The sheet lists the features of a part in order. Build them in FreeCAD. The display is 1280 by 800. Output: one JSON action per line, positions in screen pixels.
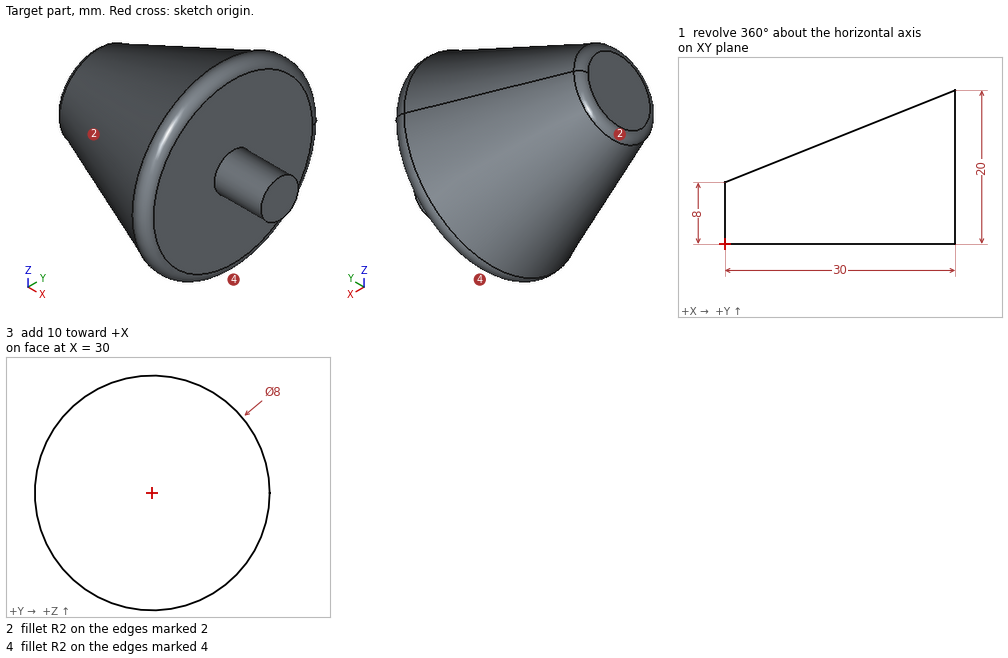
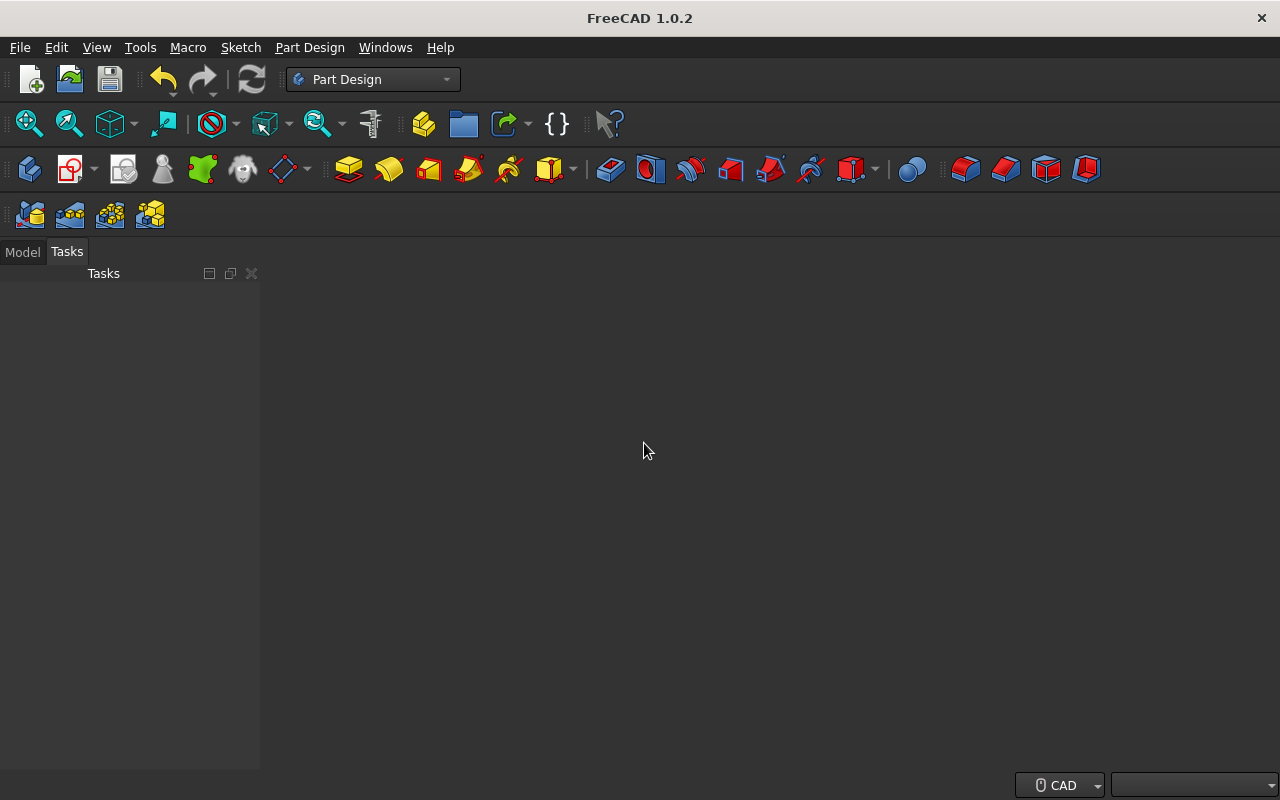
{"action": "left_click", "coordinate": [30, 80]}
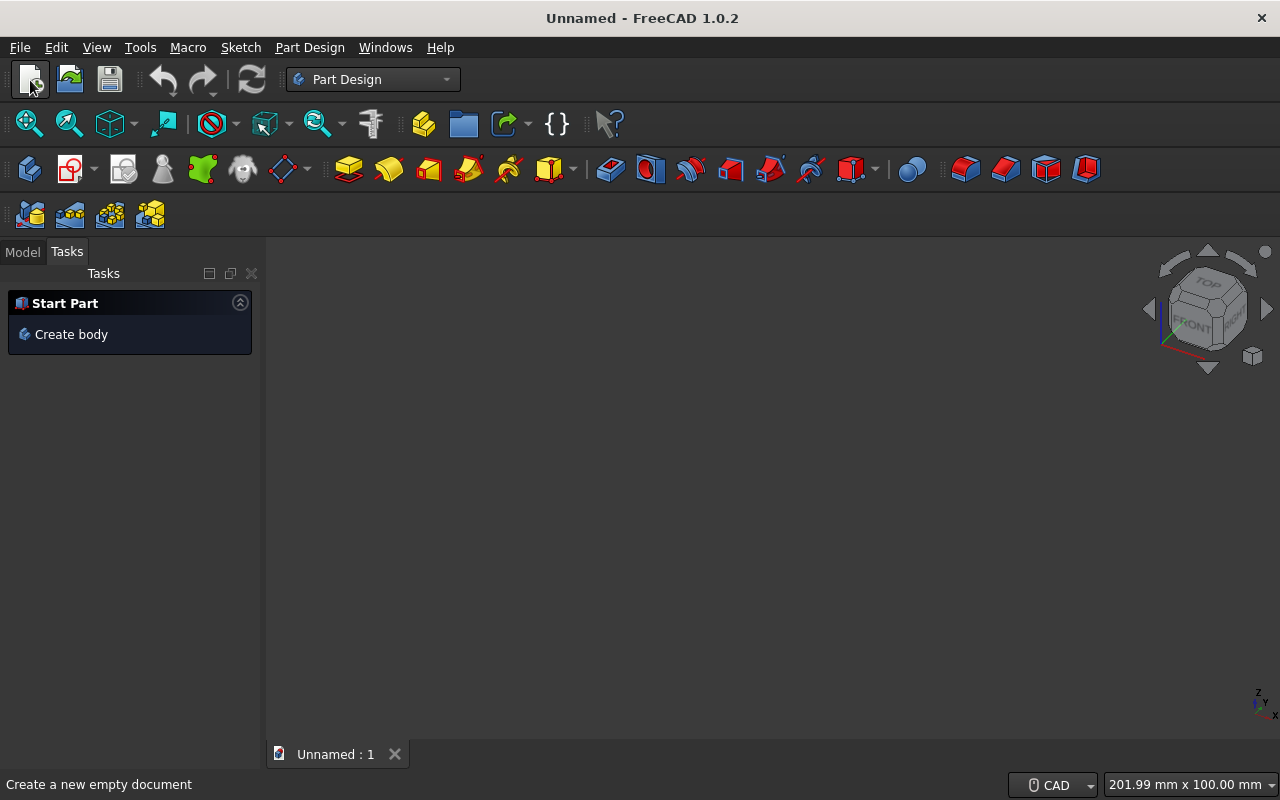
{"action": "left_click", "coordinate": [70, 170]}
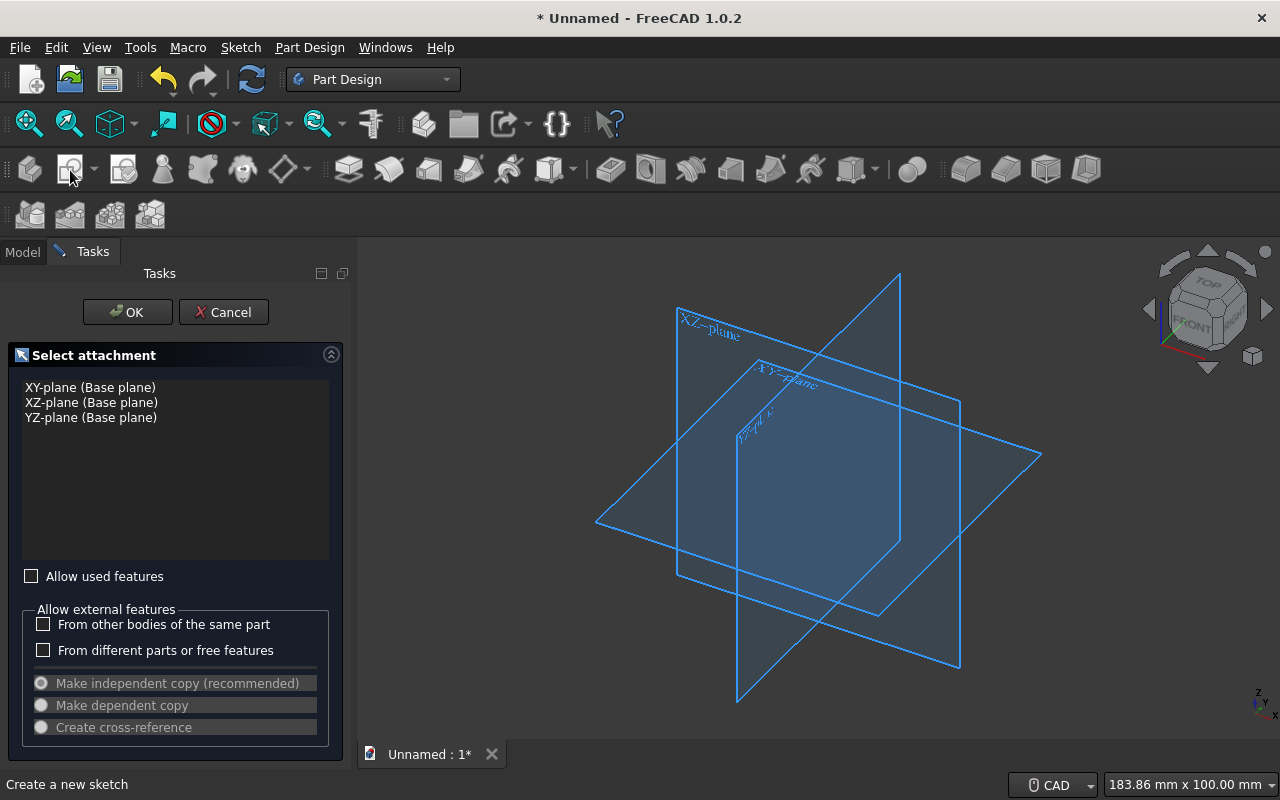
{"action": "left_click", "coordinate": [82, 388]}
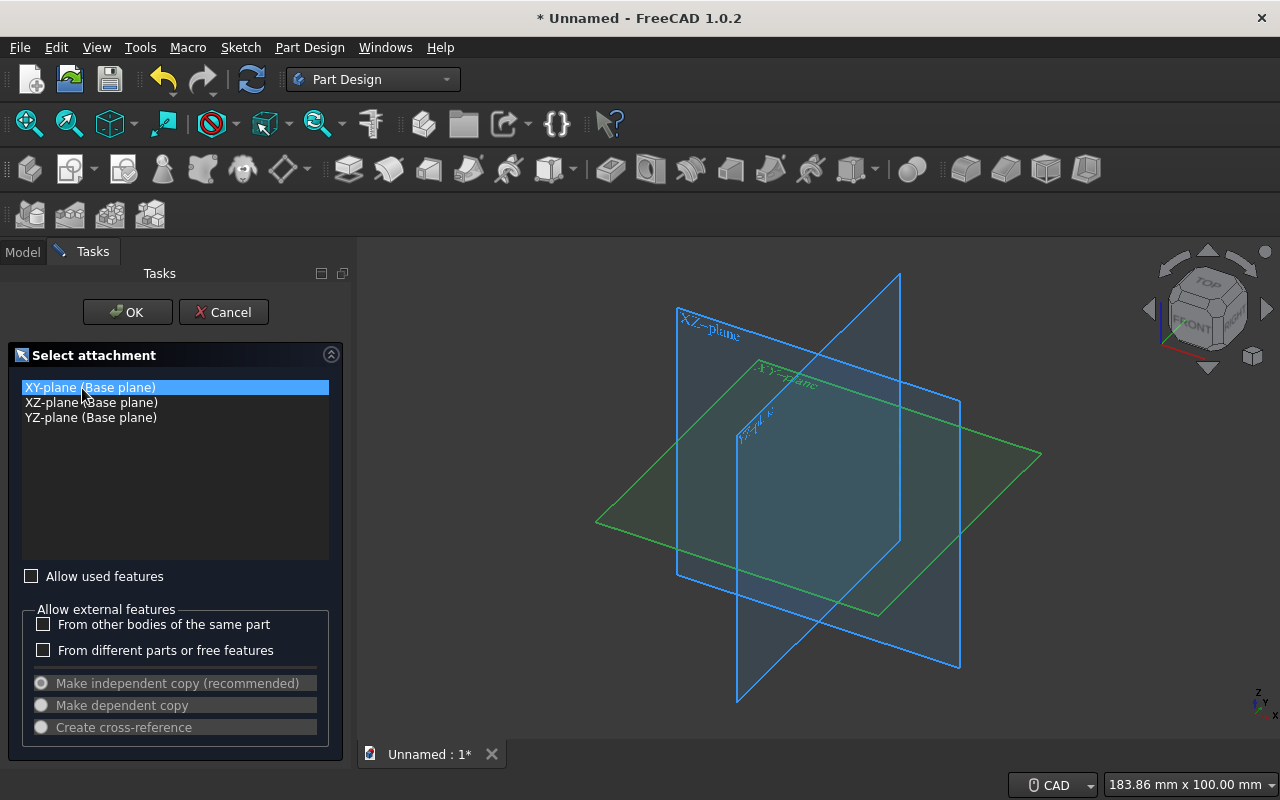
{"action": "left_click", "coordinate": [128, 312]}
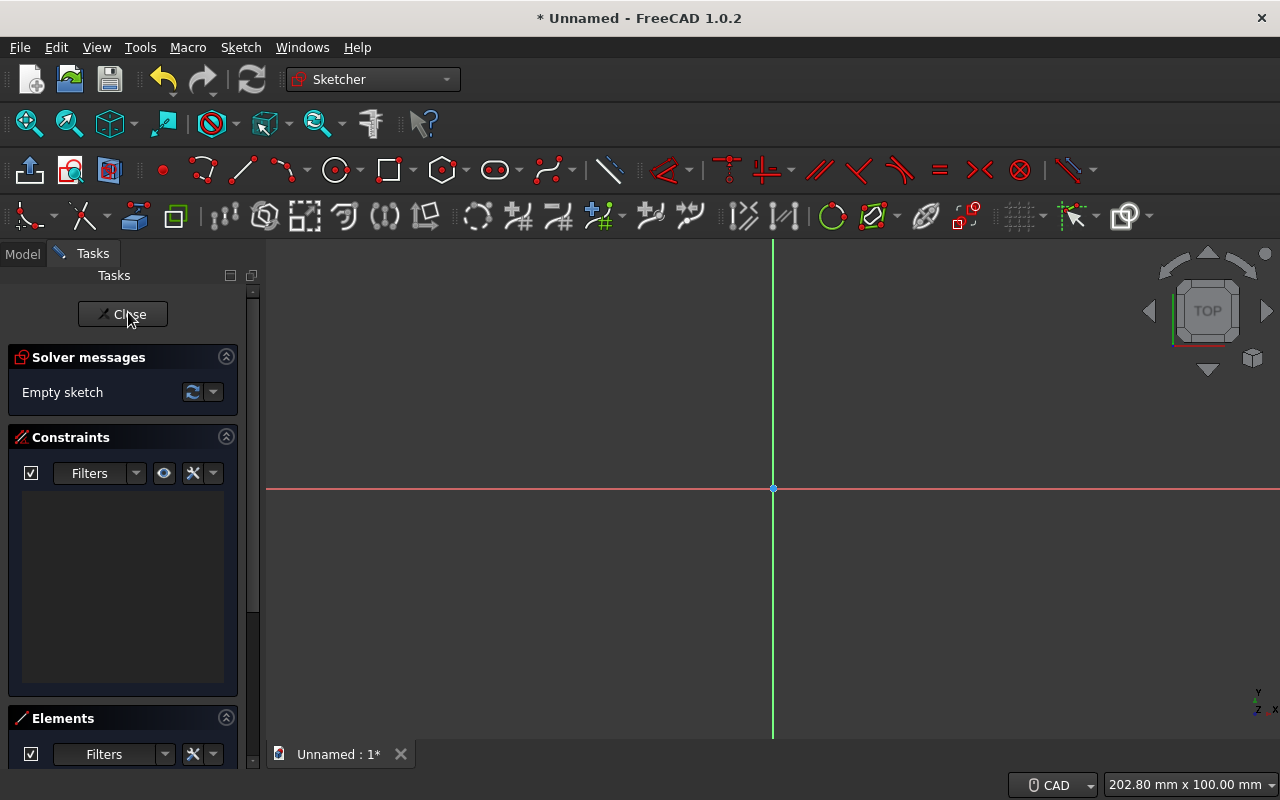
{"action": "scroll", "coordinate": [910, 417], "scroll_direction": "up", "scroll_amount": 6}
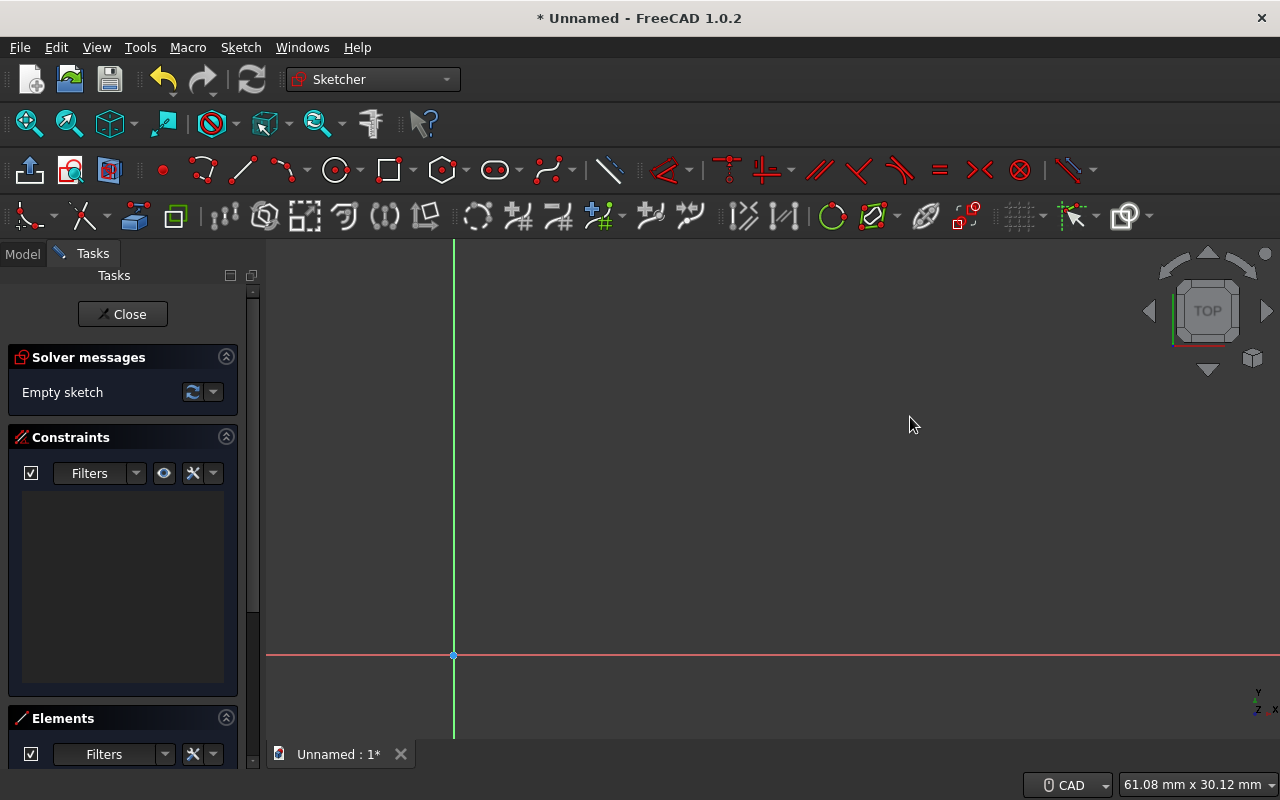
{"action": "left_click", "coordinate": [204, 170]}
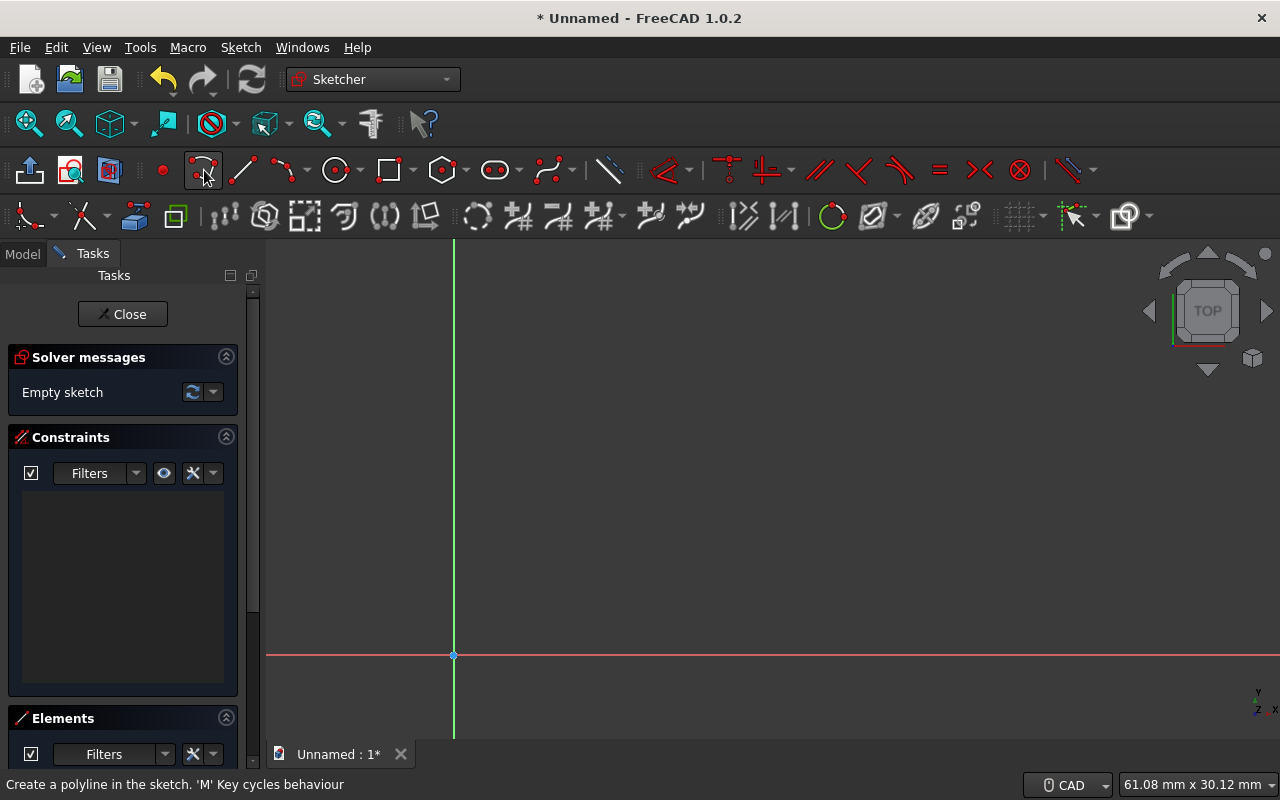
{"action": "left_click", "coordinate": [454, 655]}
{"action": "left_click", "coordinate": [952, 646]}
{"action": "left_click", "coordinate": [952, 323]}
{"action": "left_click", "coordinate": [463, 522]}
{"action": "left_click", "coordinate": [454, 655]}
{"action": "key", "text": "Escape"}
{"action": "key", "text": "Escape"}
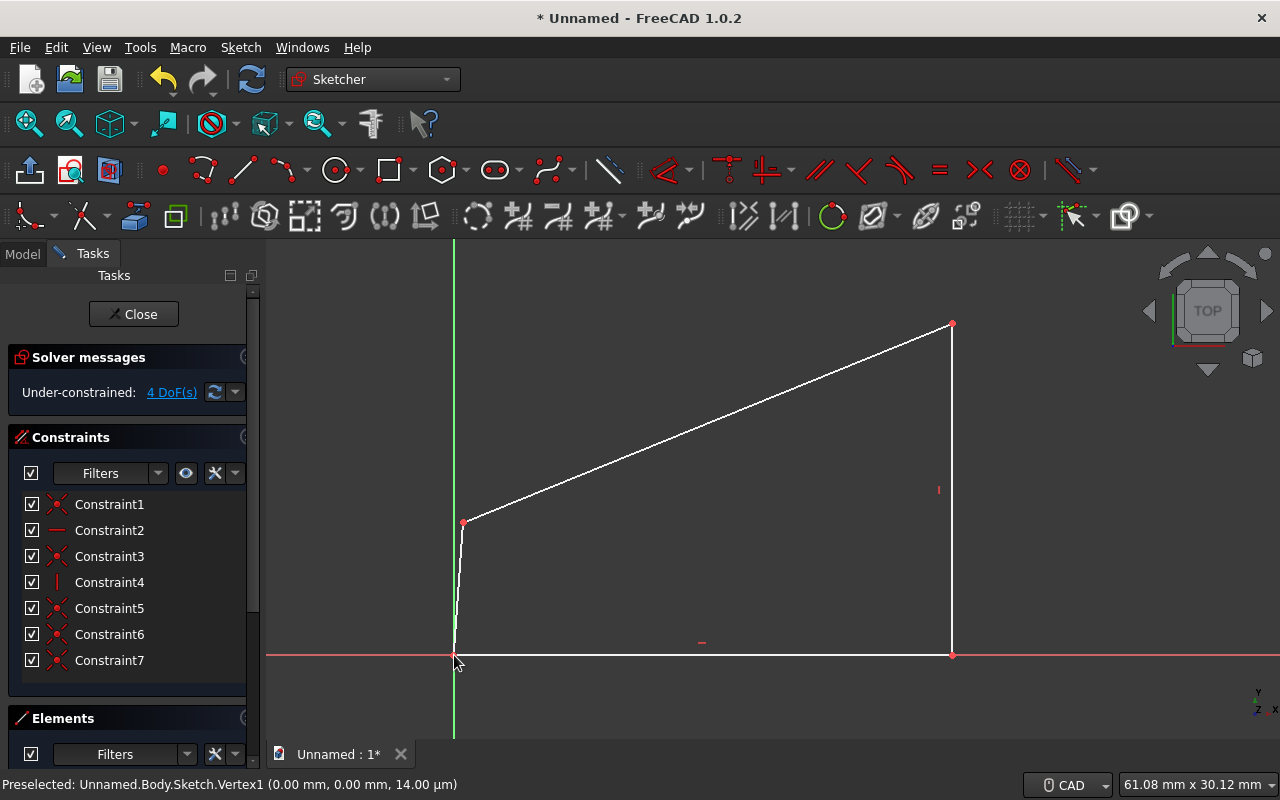
{"action": "left_click", "coordinate": [456, 616]}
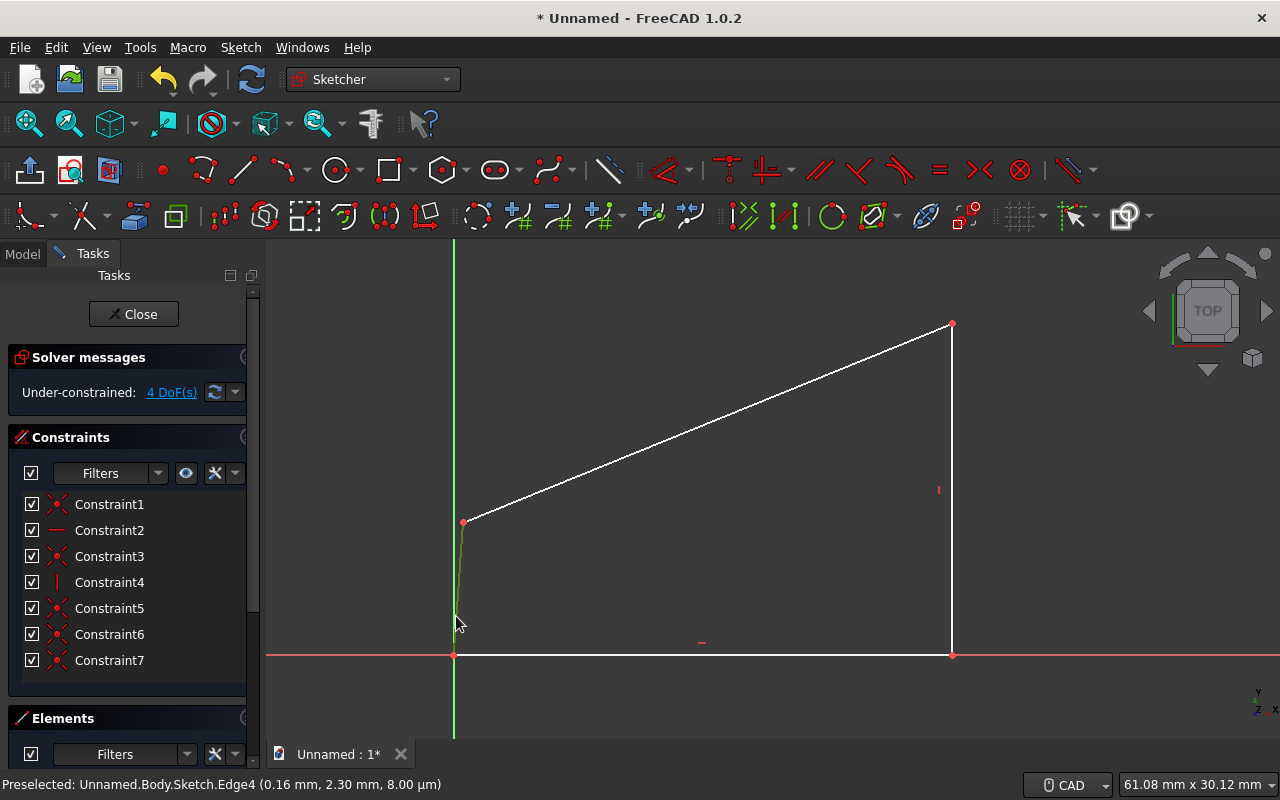
{"action": "key", "text": "v"}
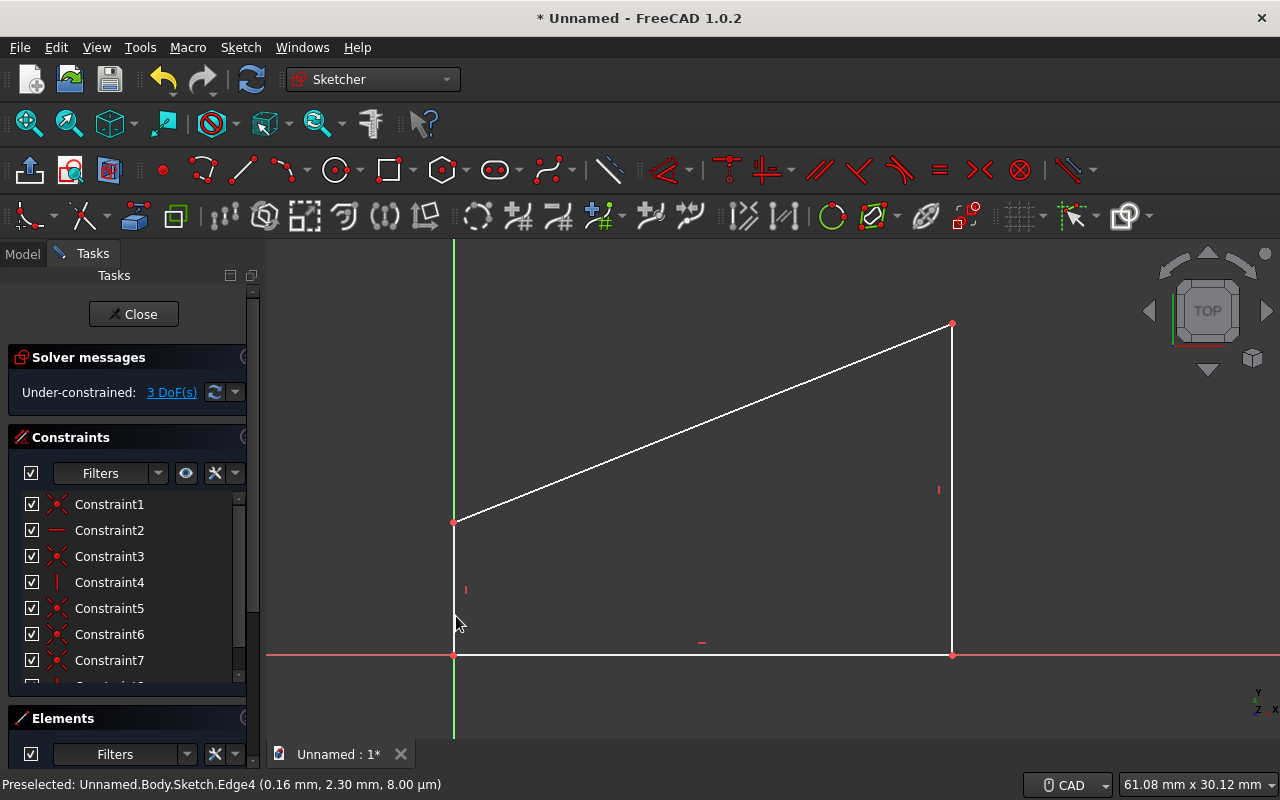
{"action": "left_click", "coordinate": [664, 170]}